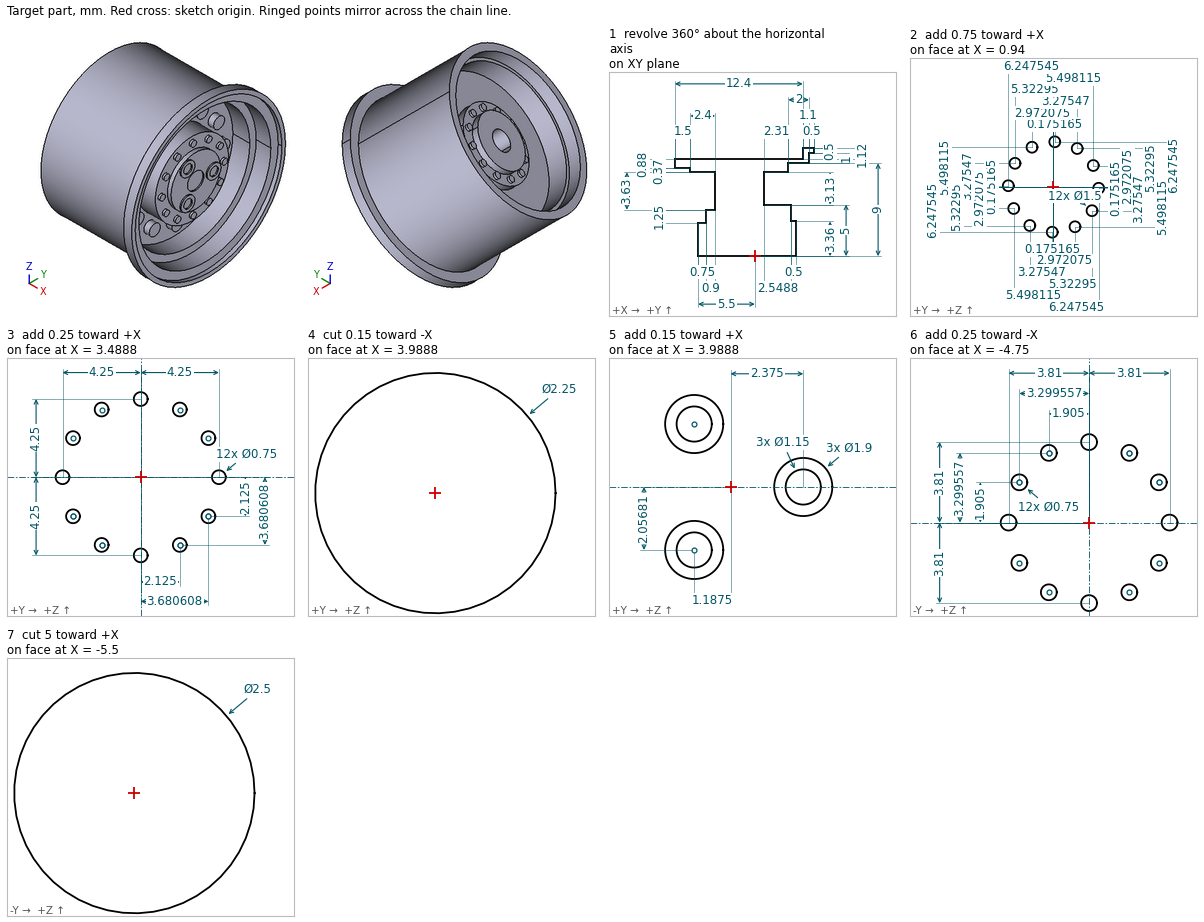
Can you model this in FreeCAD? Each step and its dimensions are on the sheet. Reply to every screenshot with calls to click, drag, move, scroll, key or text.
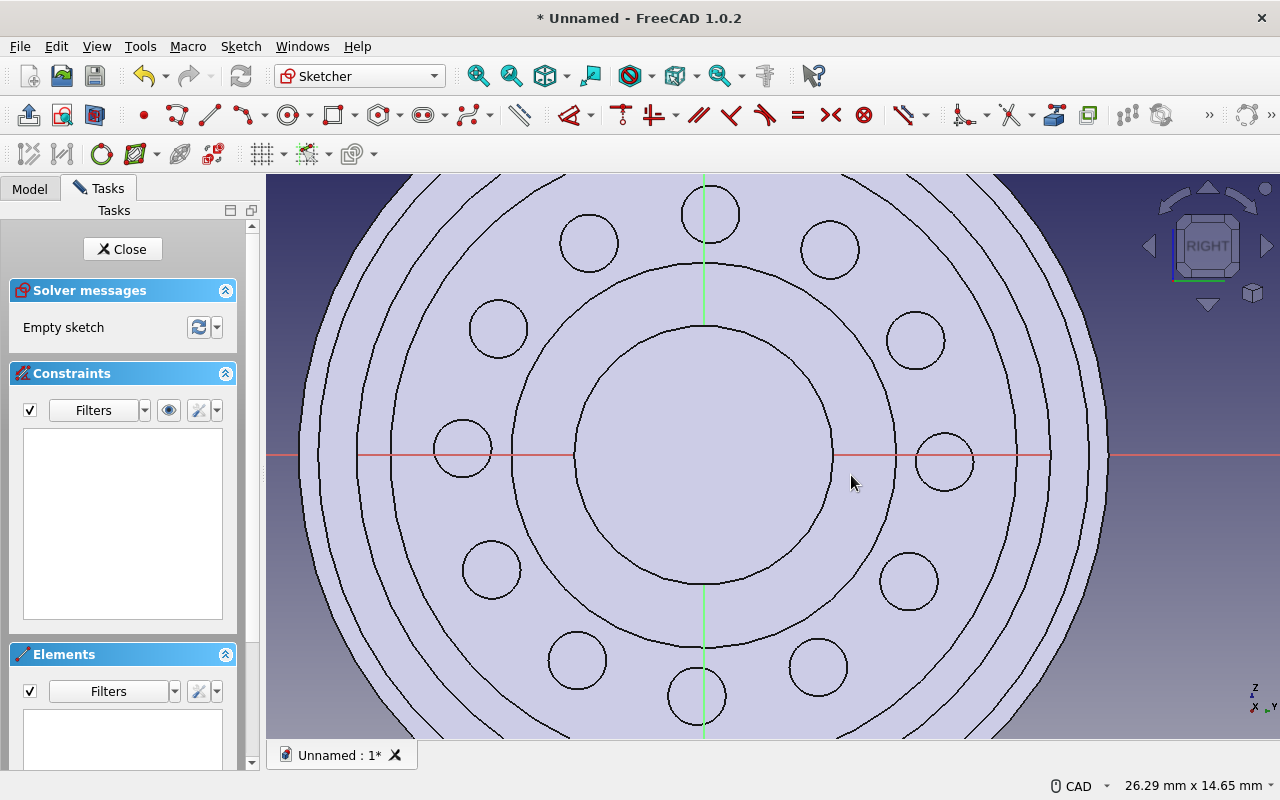
click(288, 116)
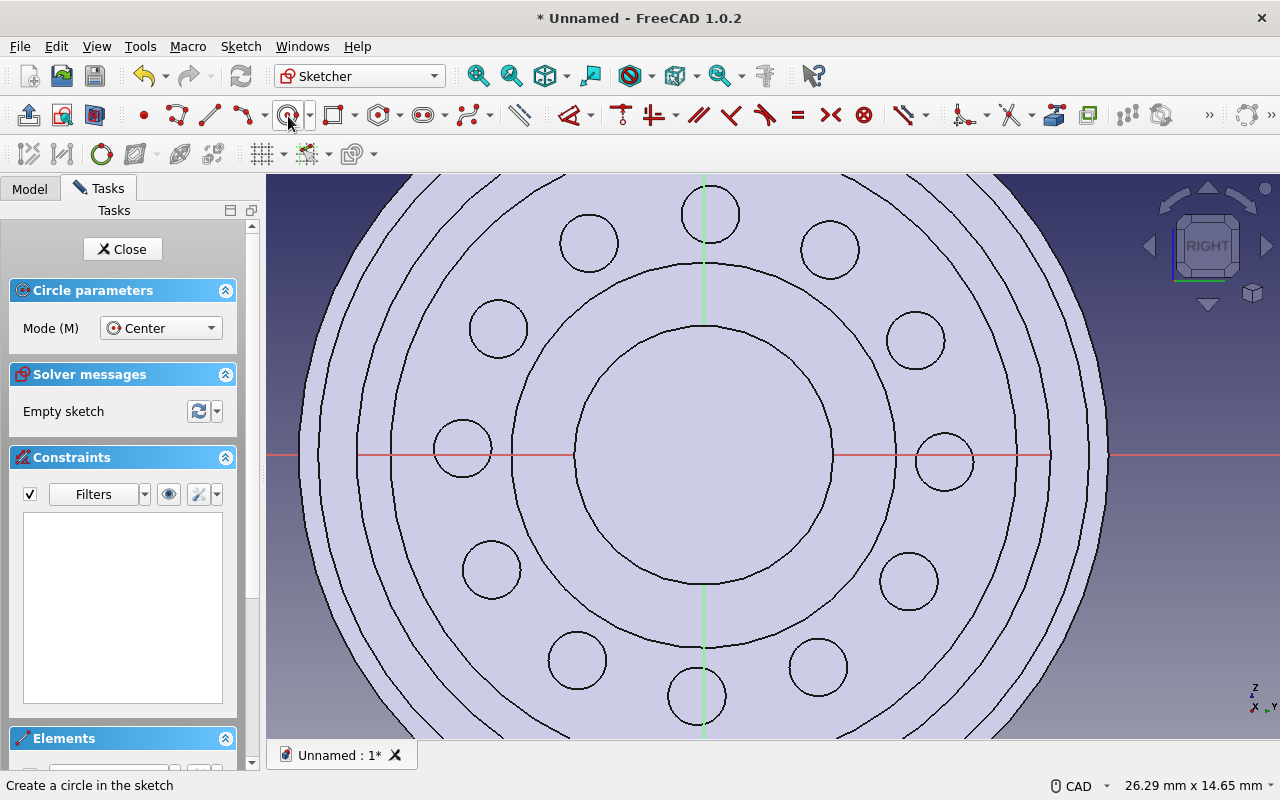
scroll(868, 455, up, 3)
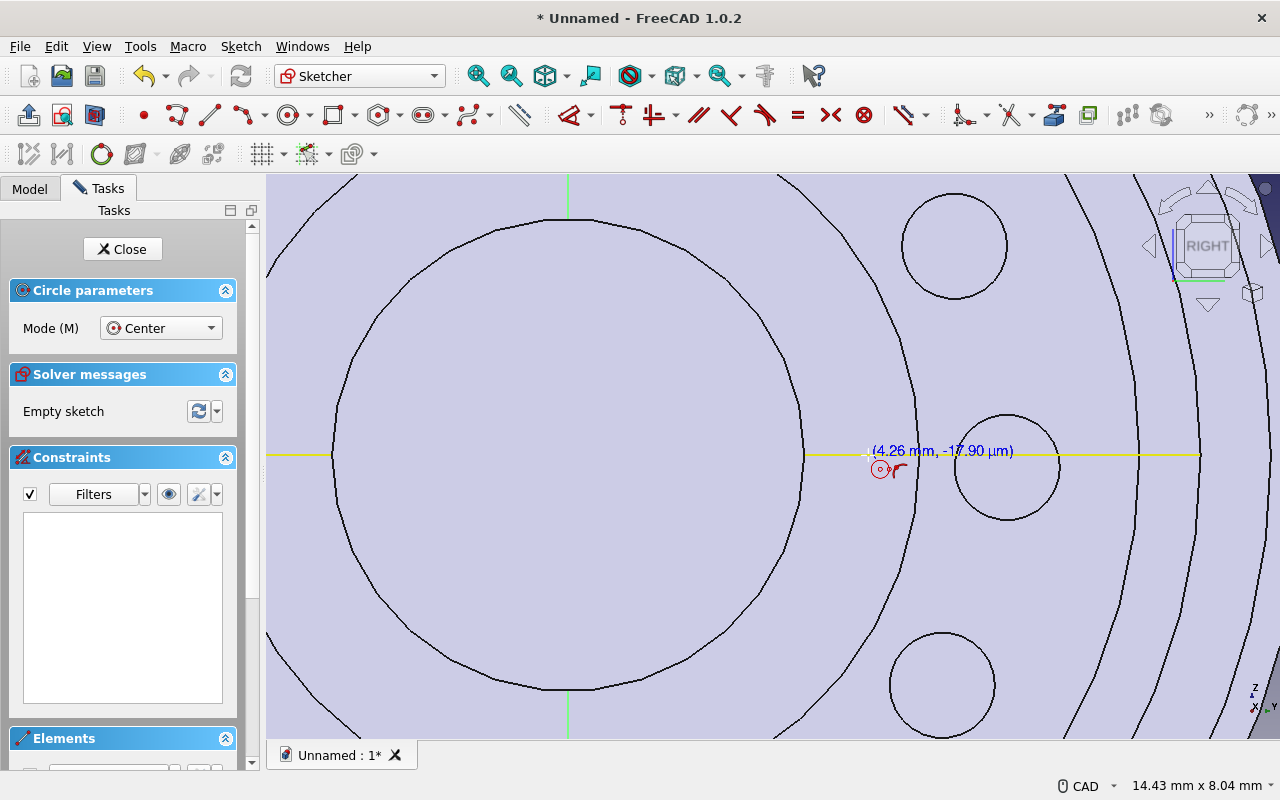
click(867, 455)
move(885, 437)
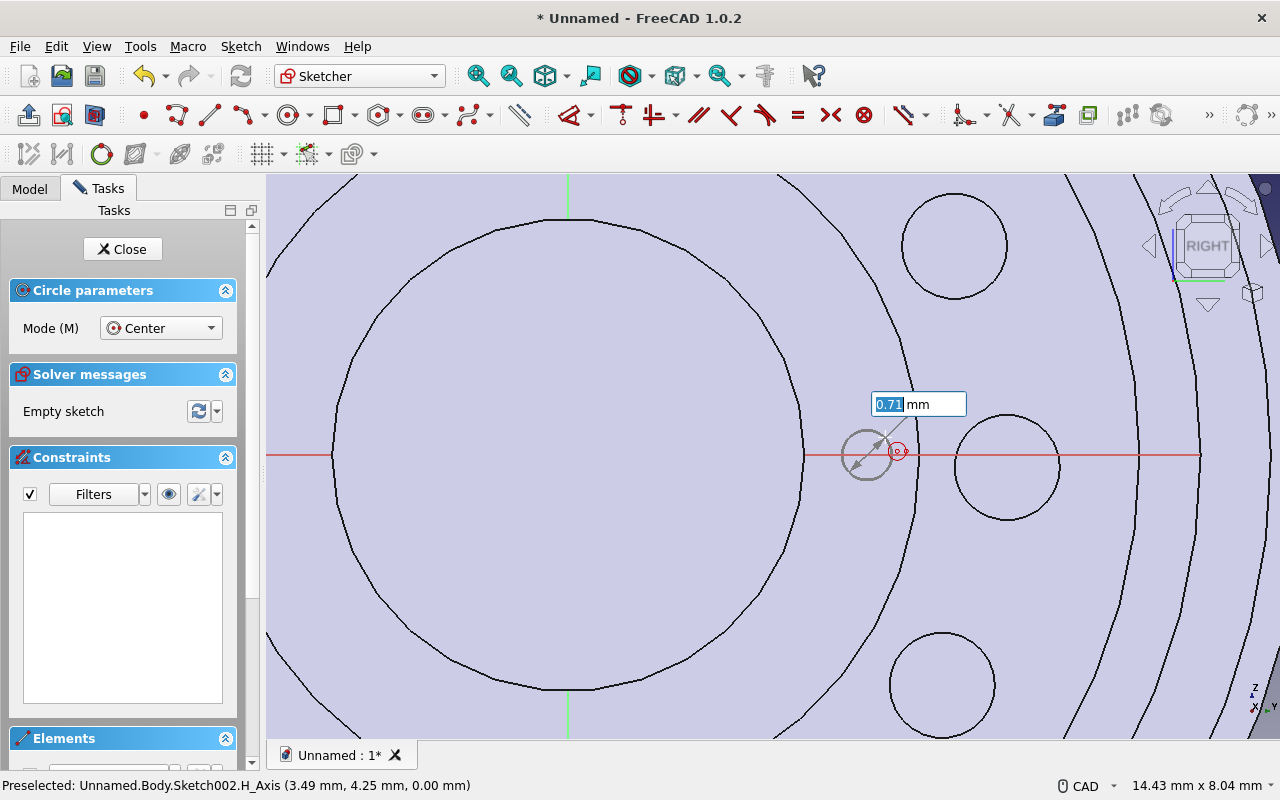
text(0.75)
key(Return)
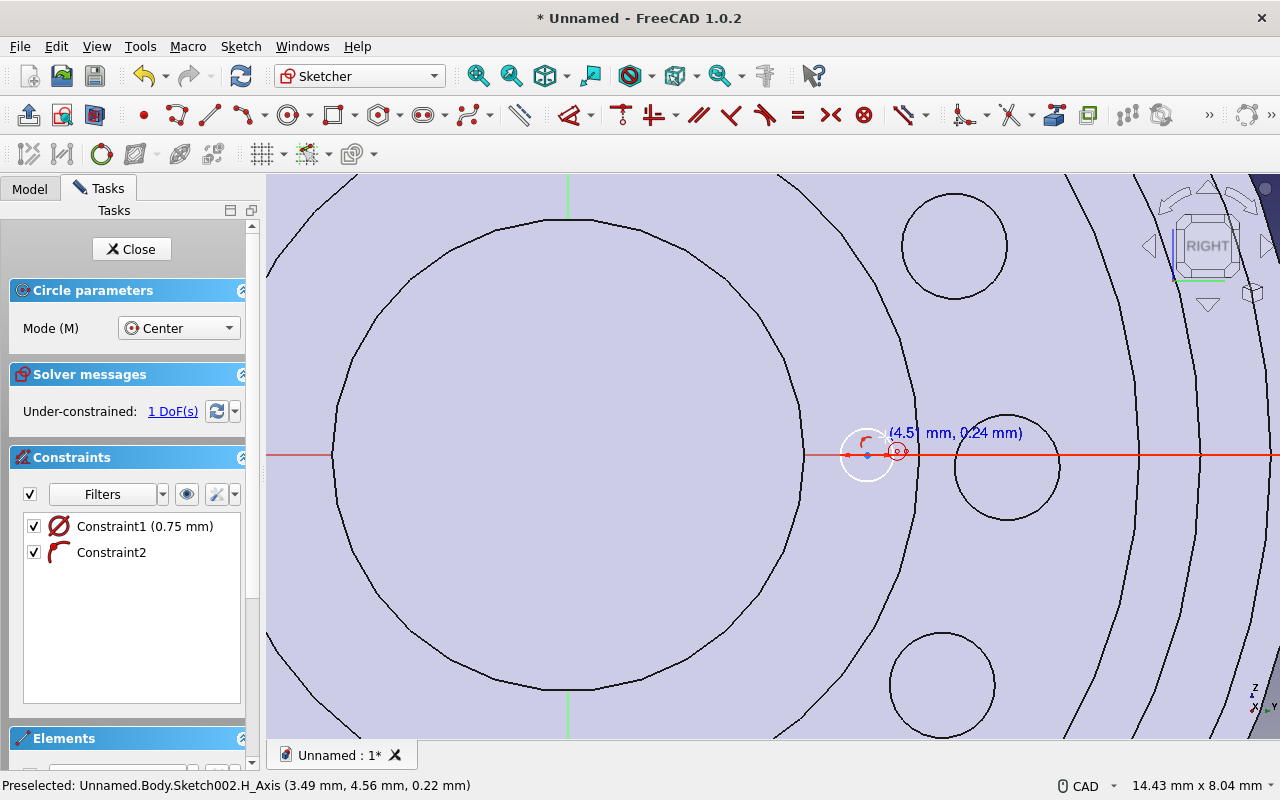
click(827, 604)
move(845, 586)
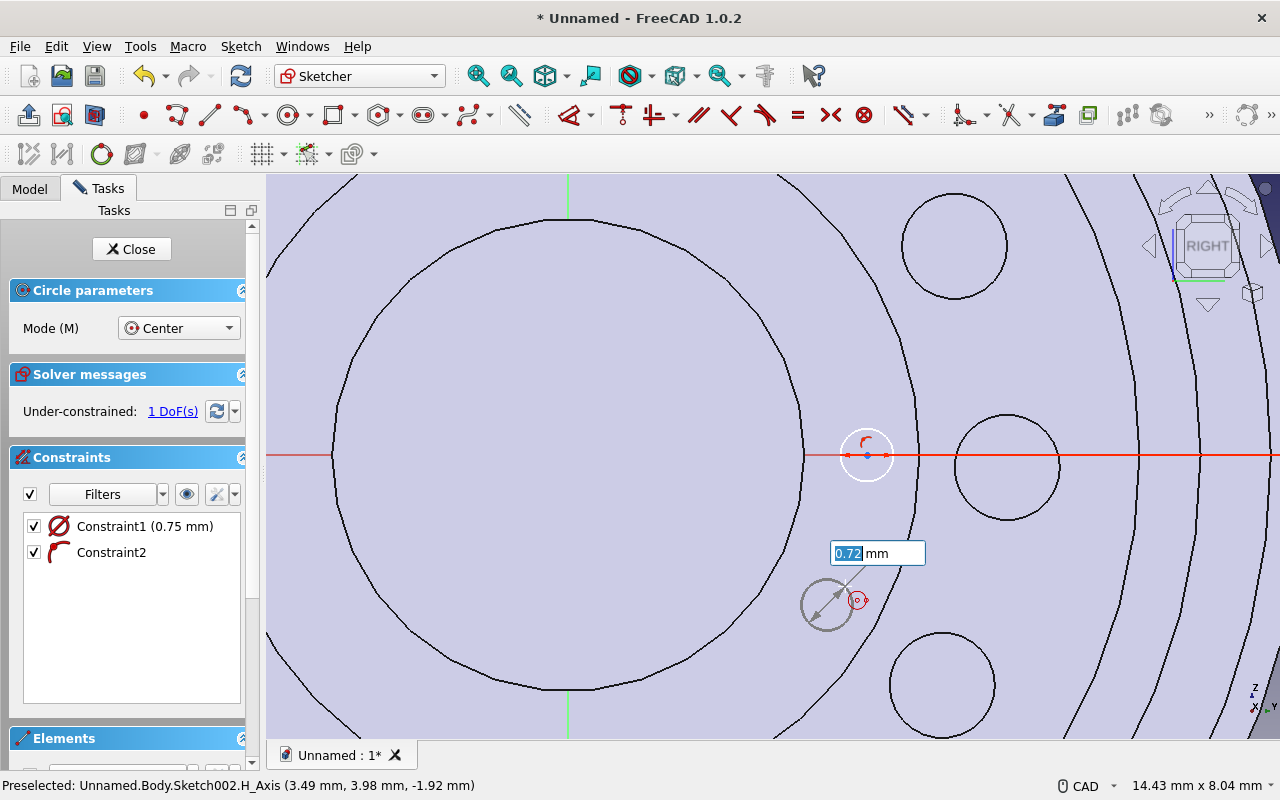
text(0.75)
key(Return)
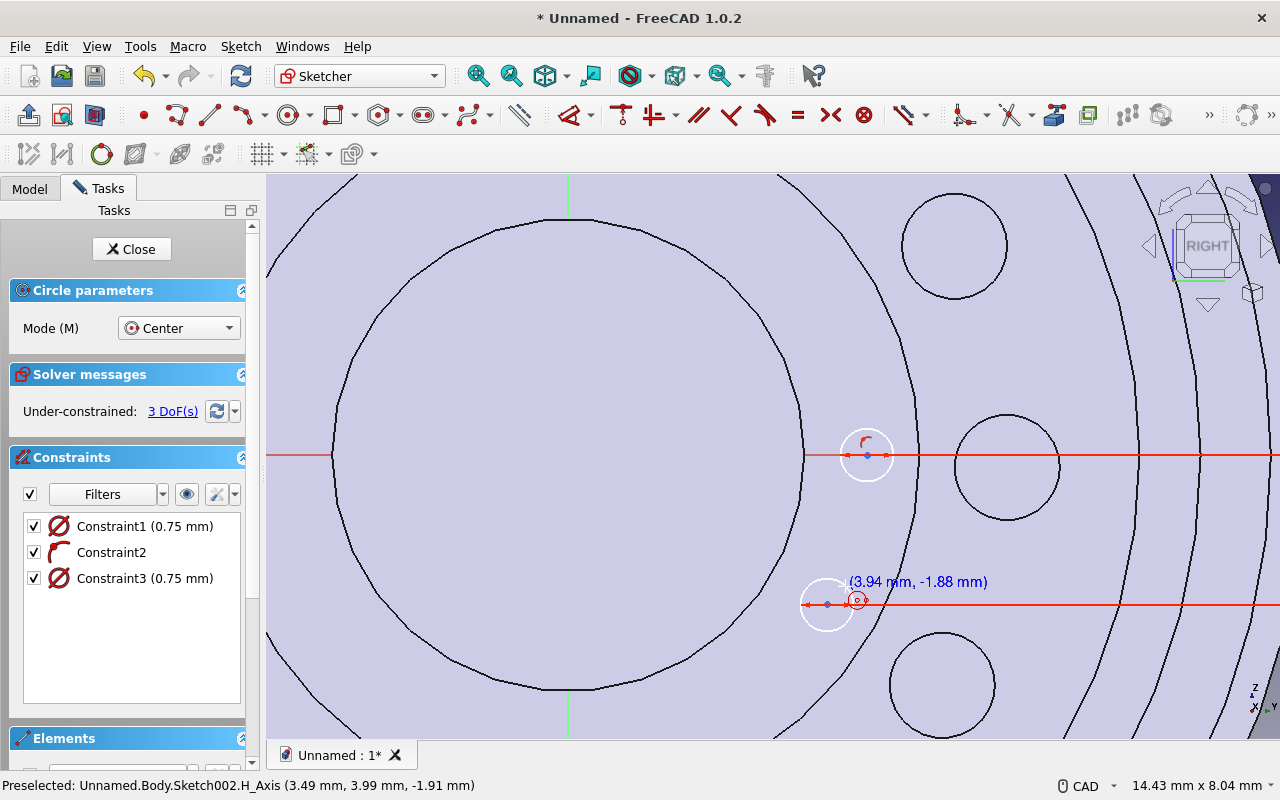
scroll(870, 458, down, 3)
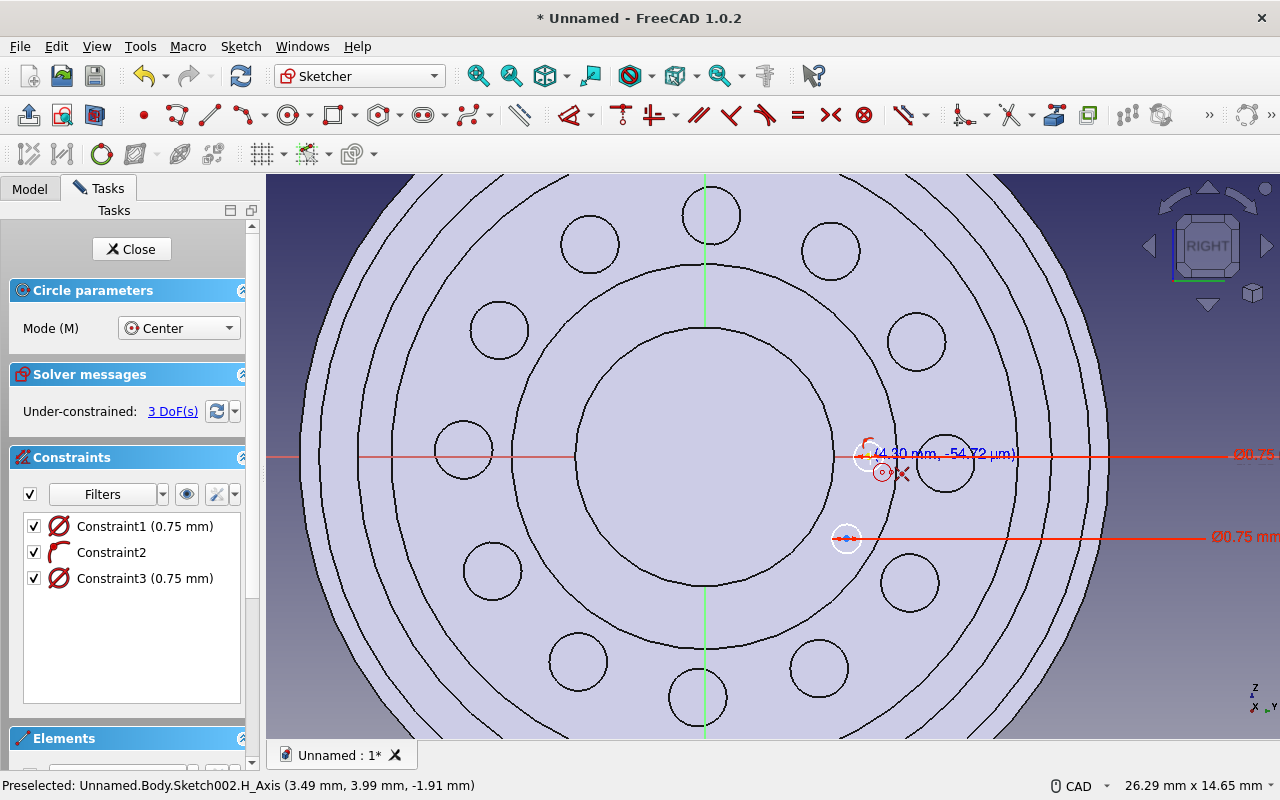
scroll(787, 599, up, 3)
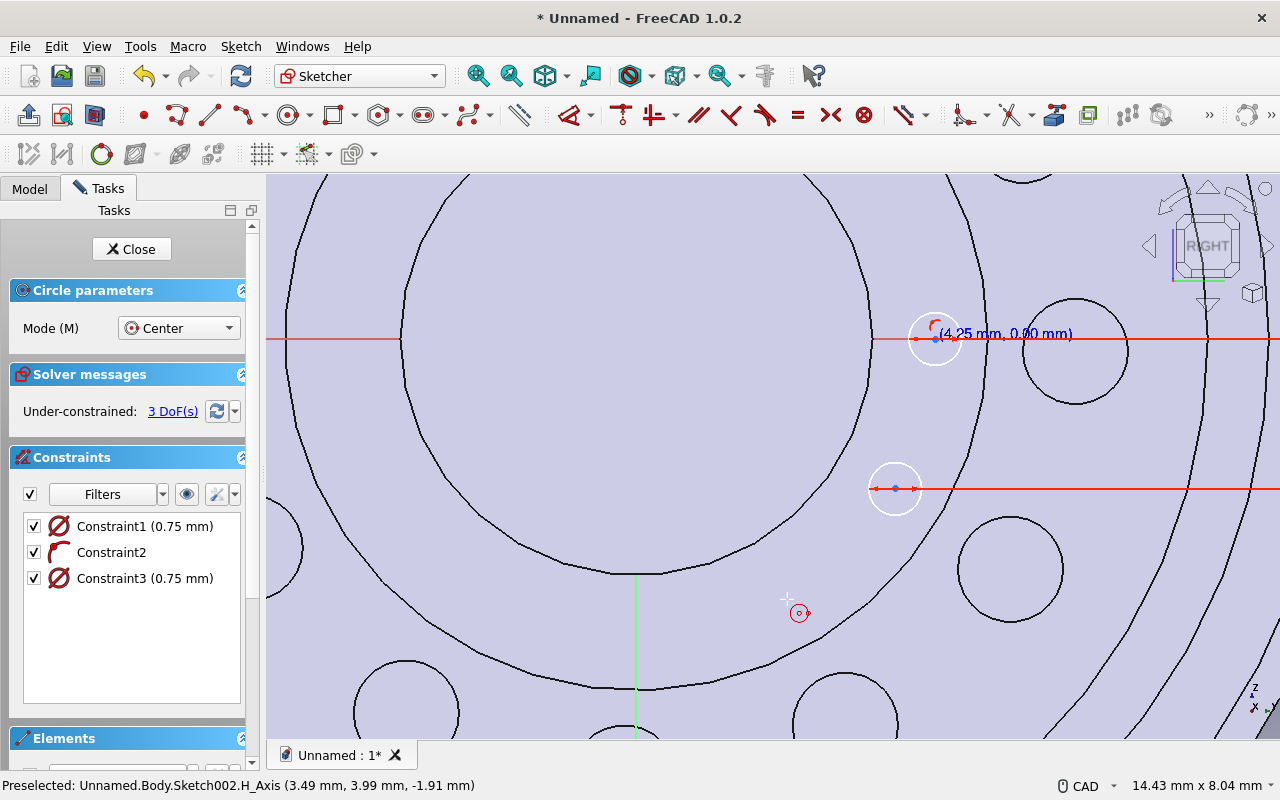
click(786, 598)
move(804, 579)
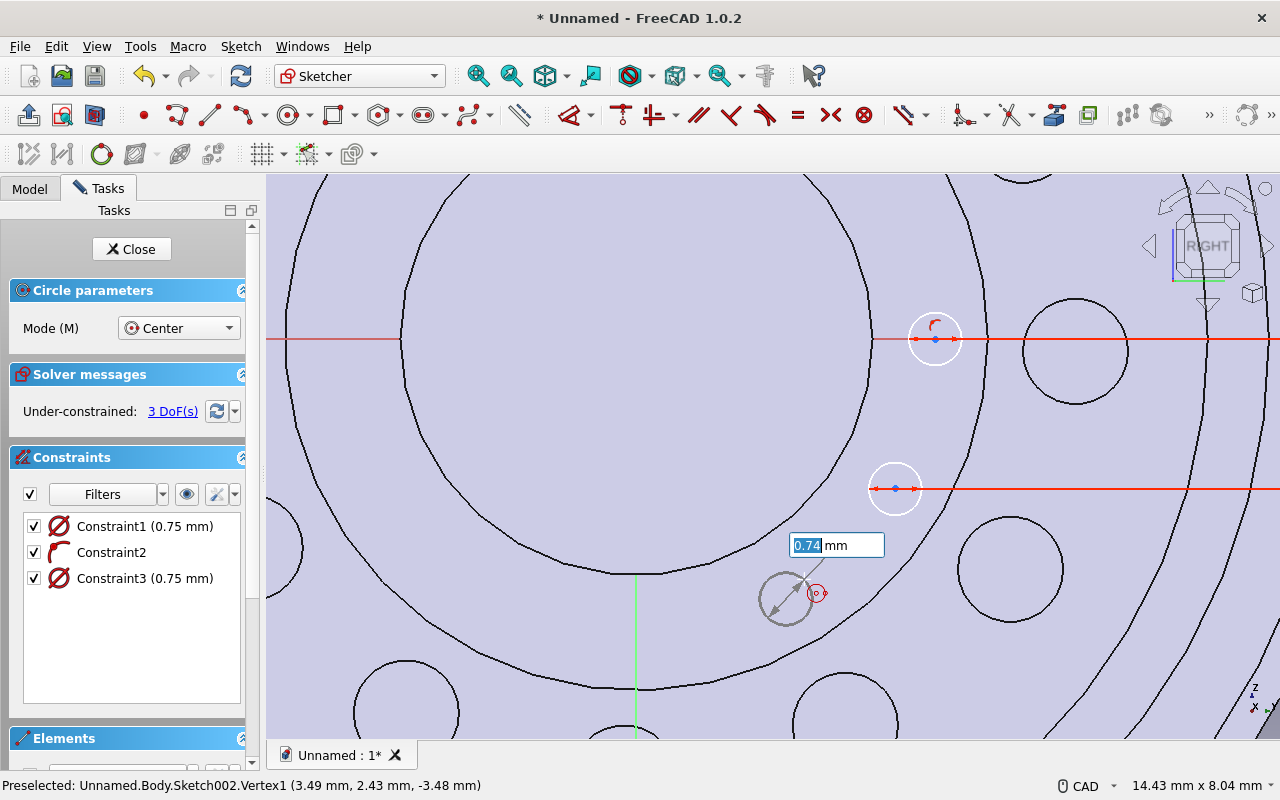
text(0.75)
key(Return)